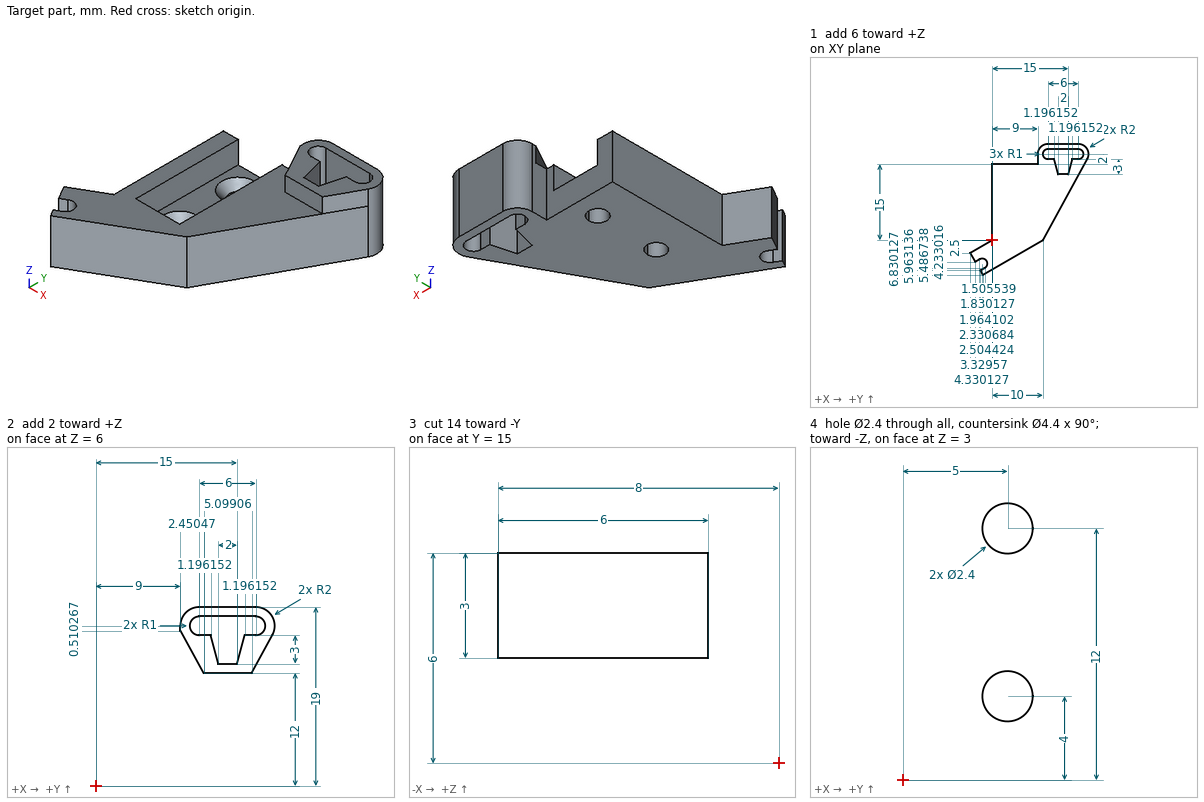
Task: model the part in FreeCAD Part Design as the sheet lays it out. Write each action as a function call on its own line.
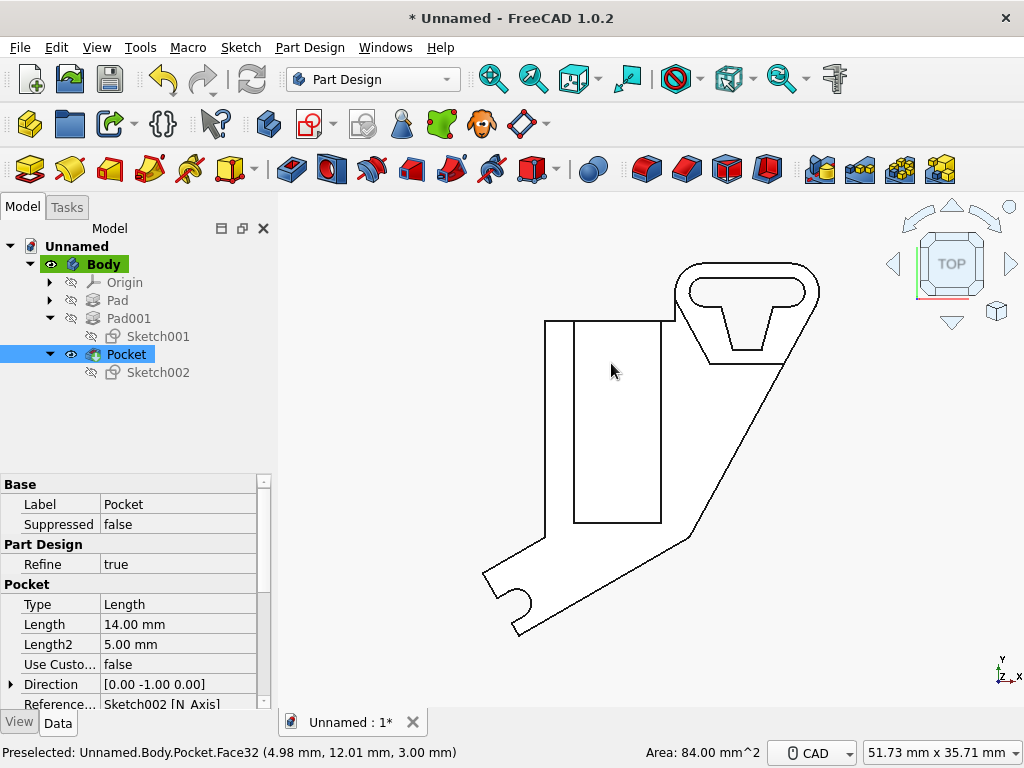
click(310, 124)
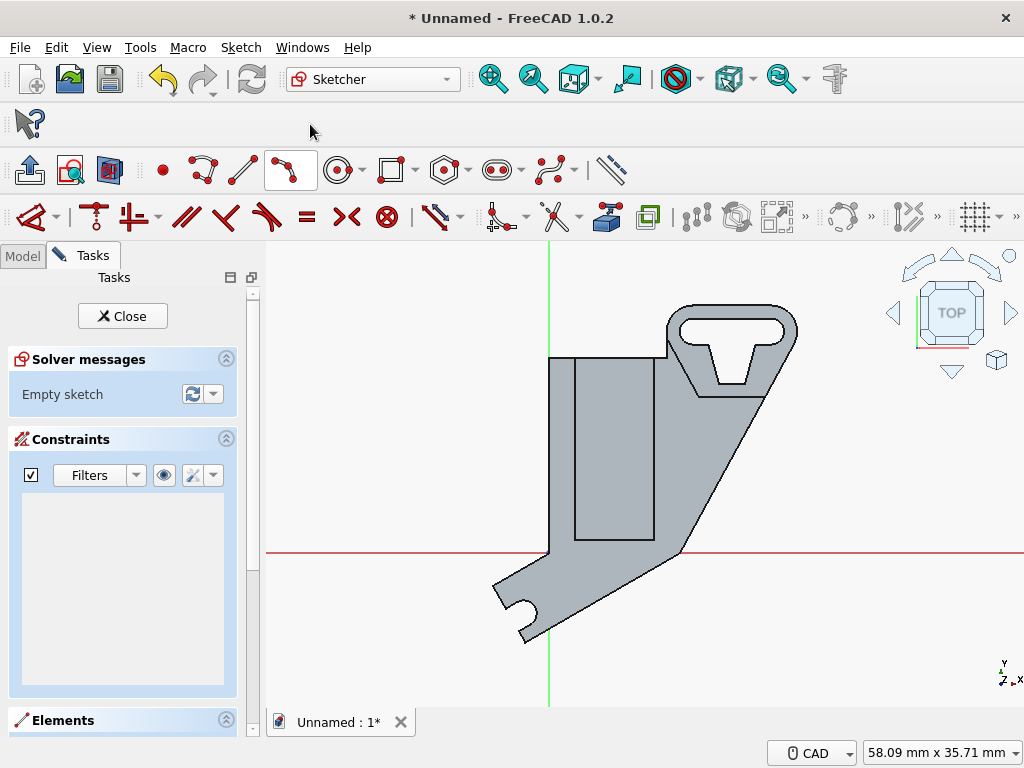
click(110, 170)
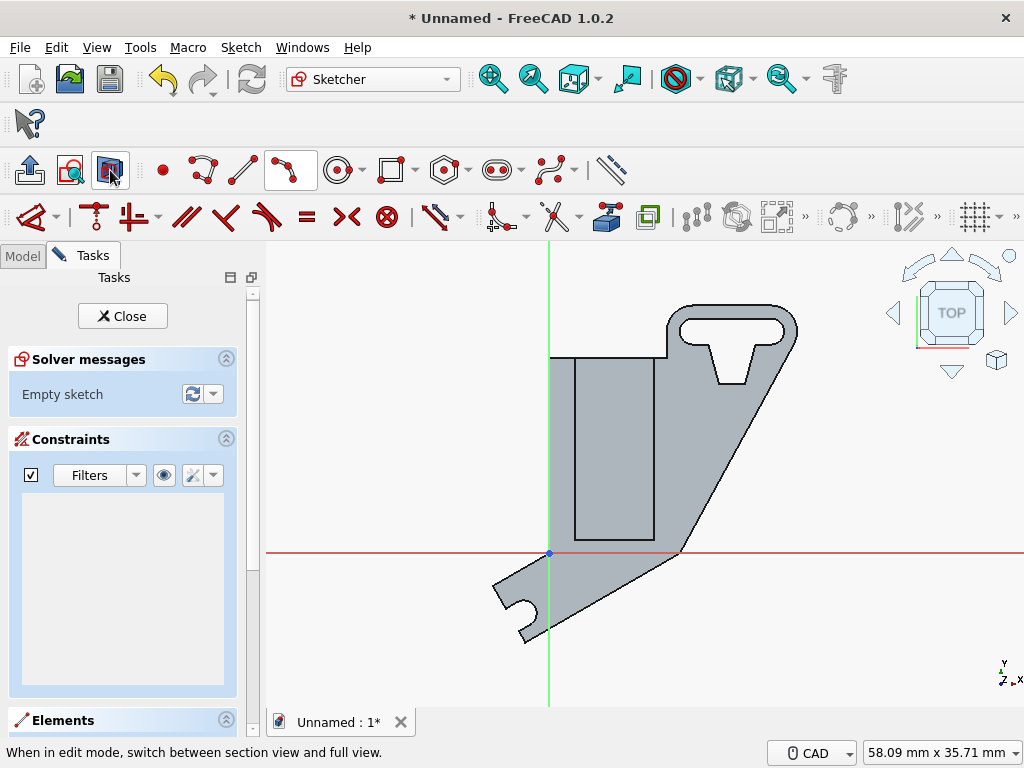
scroll(606, 459, up, 3)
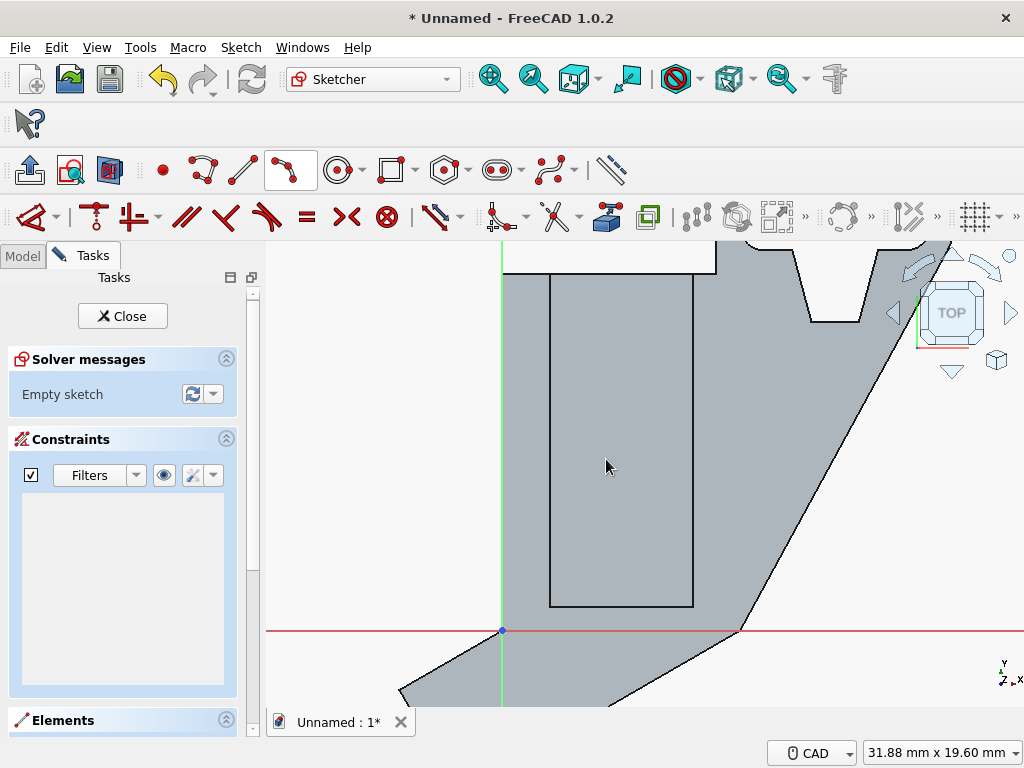
click(338, 170)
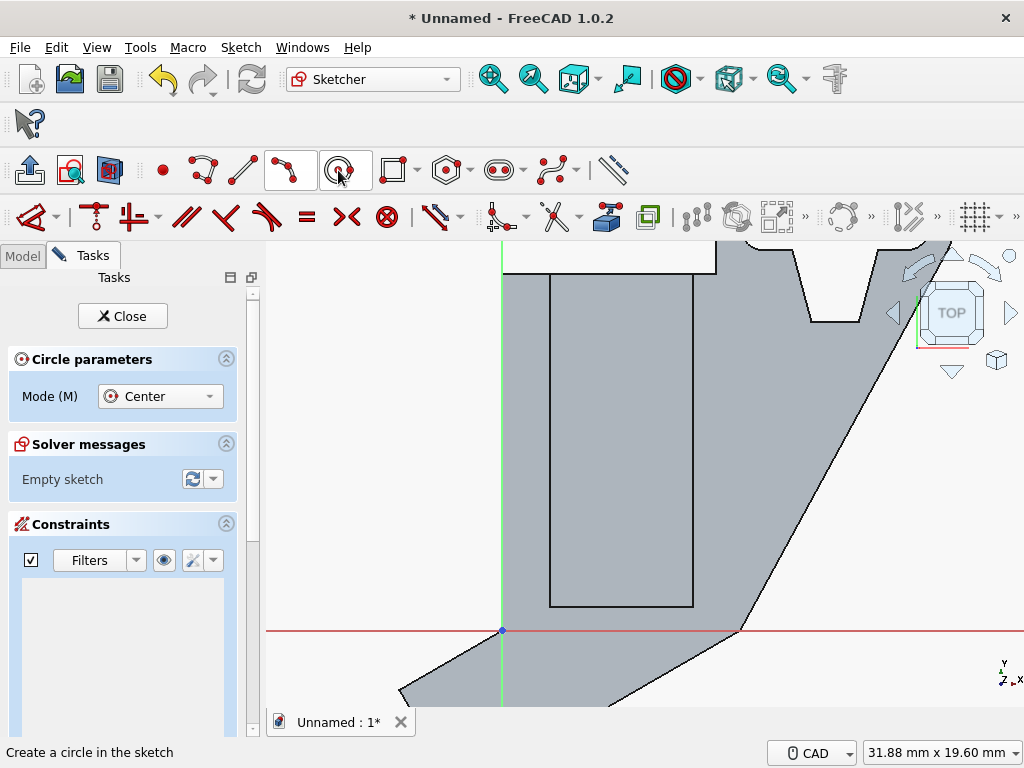
click(621, 345)
click(641, 325)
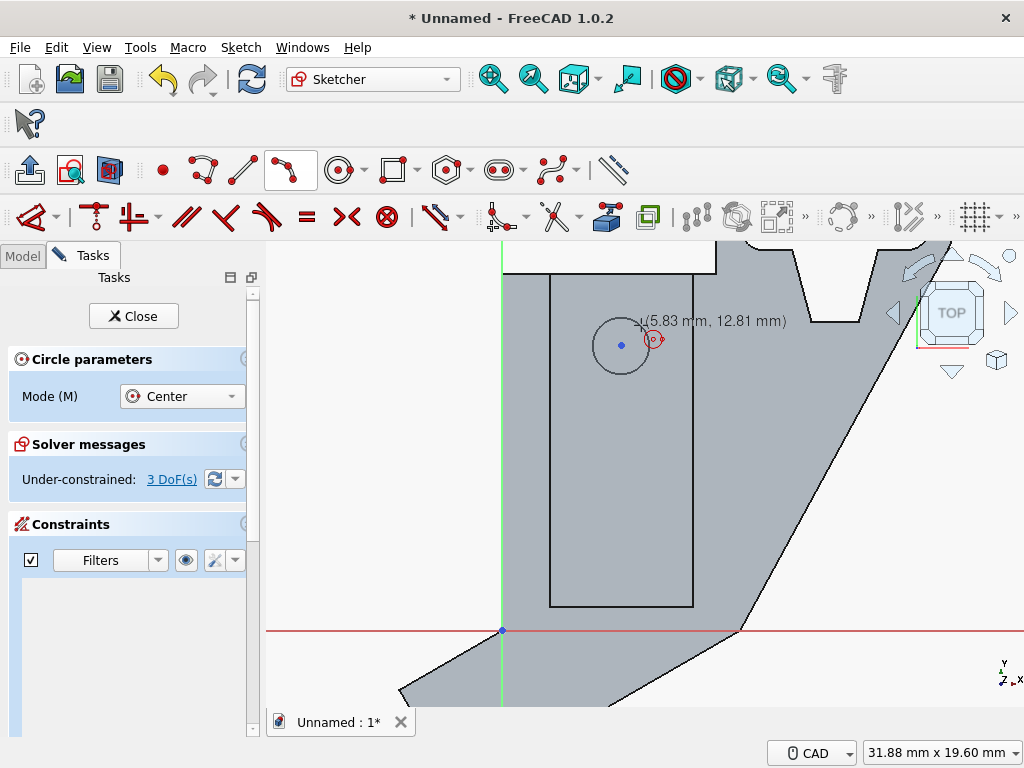
click(621, 536)
click(641, 515)
key(Escape)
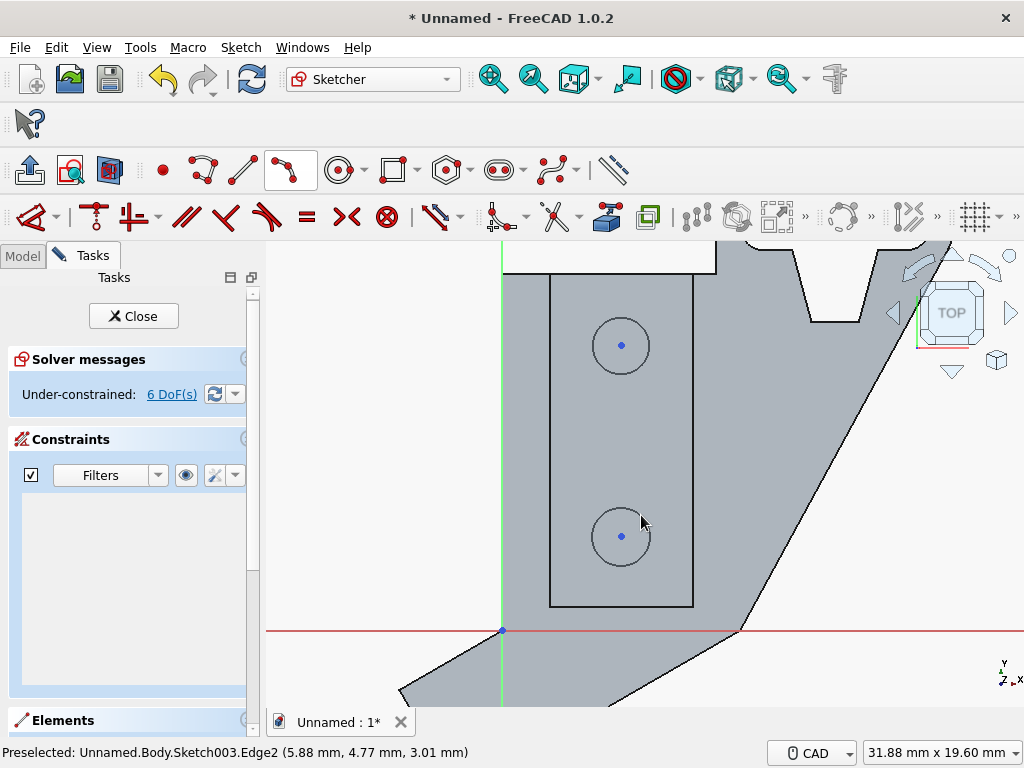
click(641, 326)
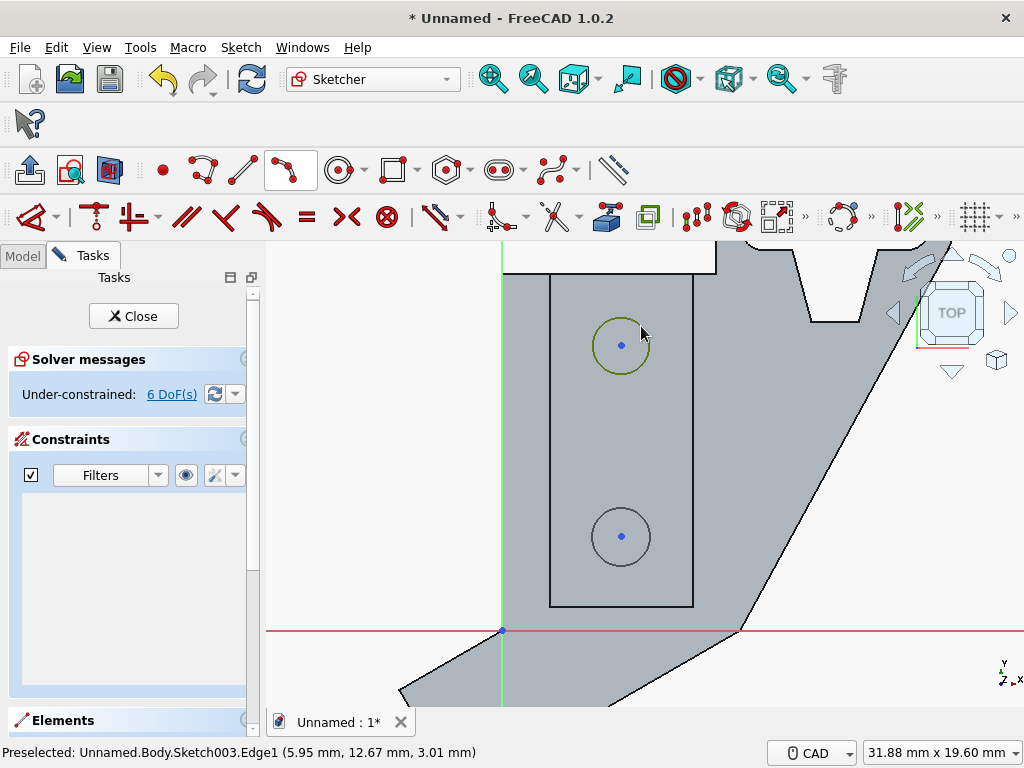
click(641, 516)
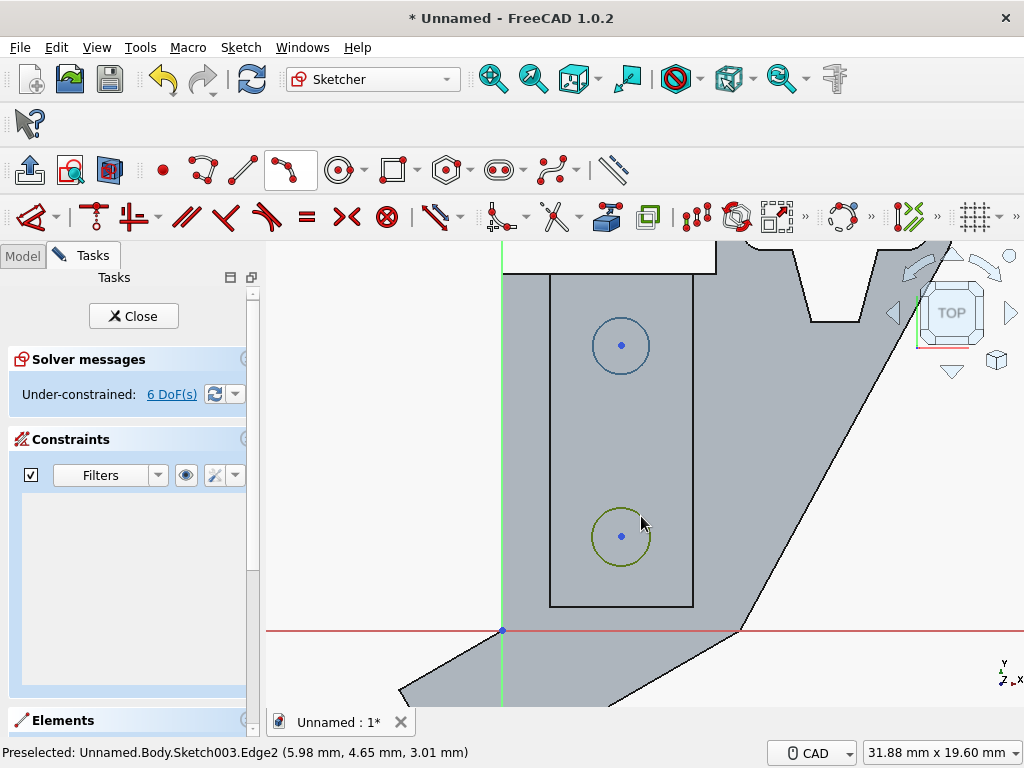
key(e)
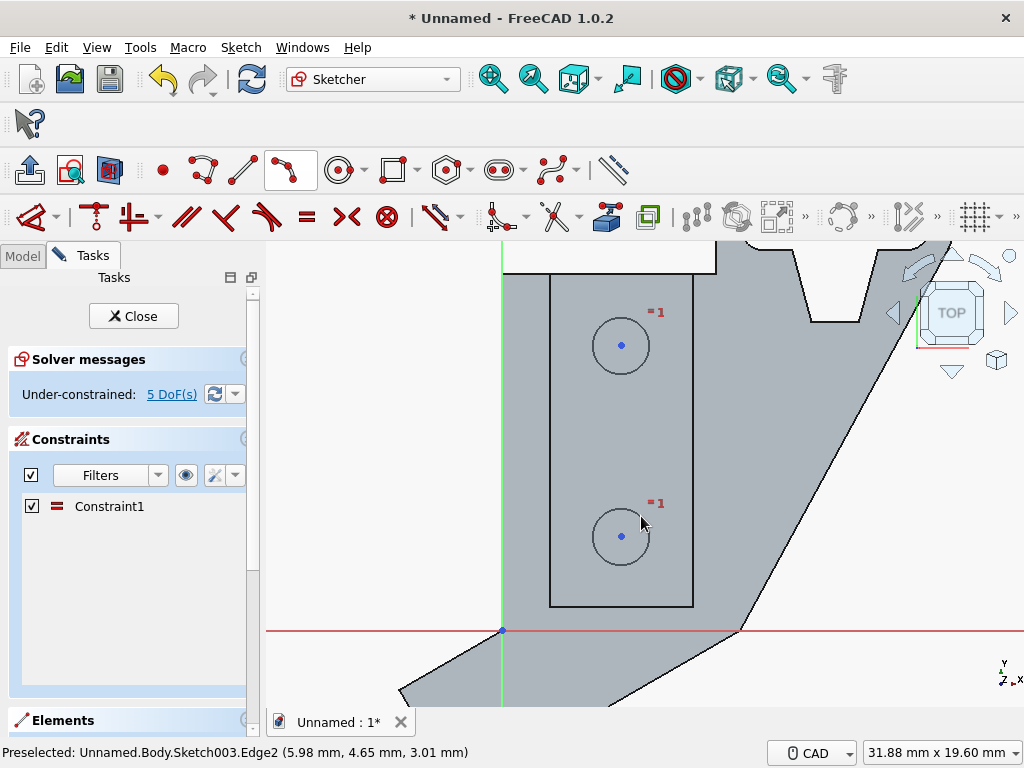
click(621, 346)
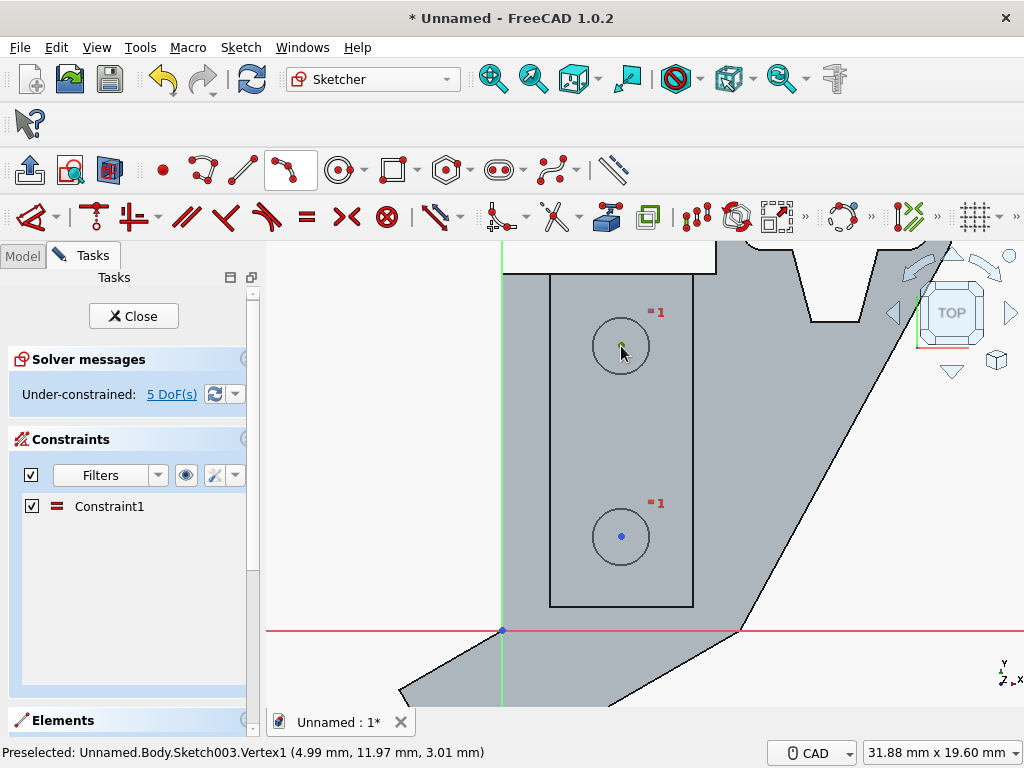
click(621, 537)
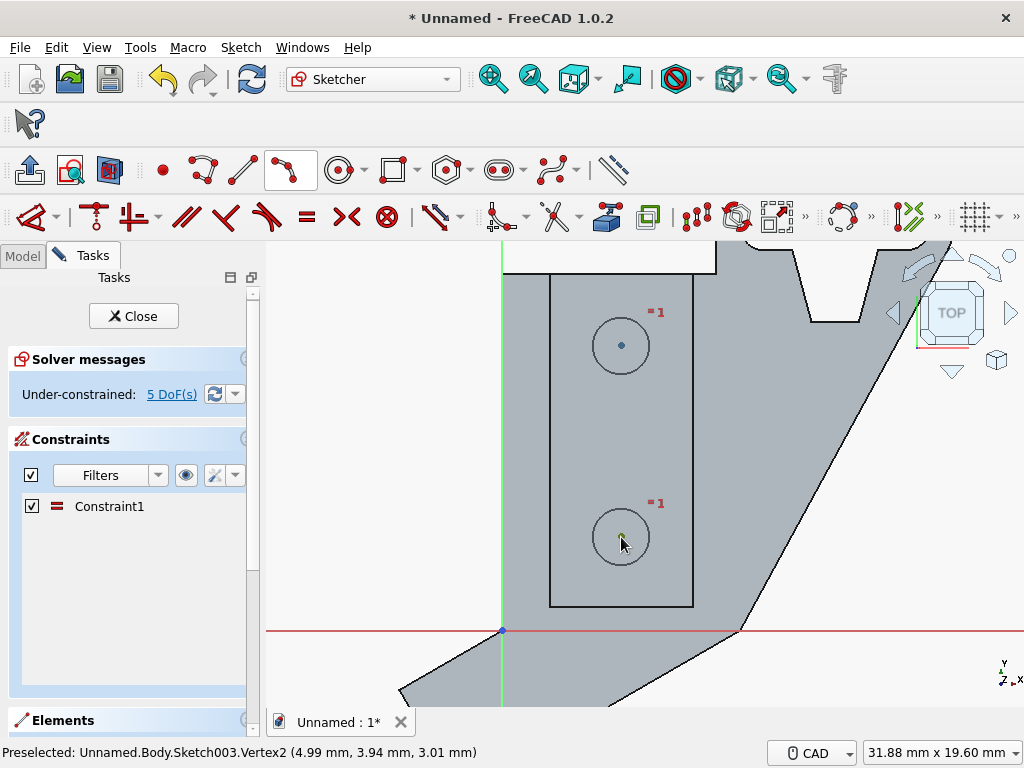
key(v)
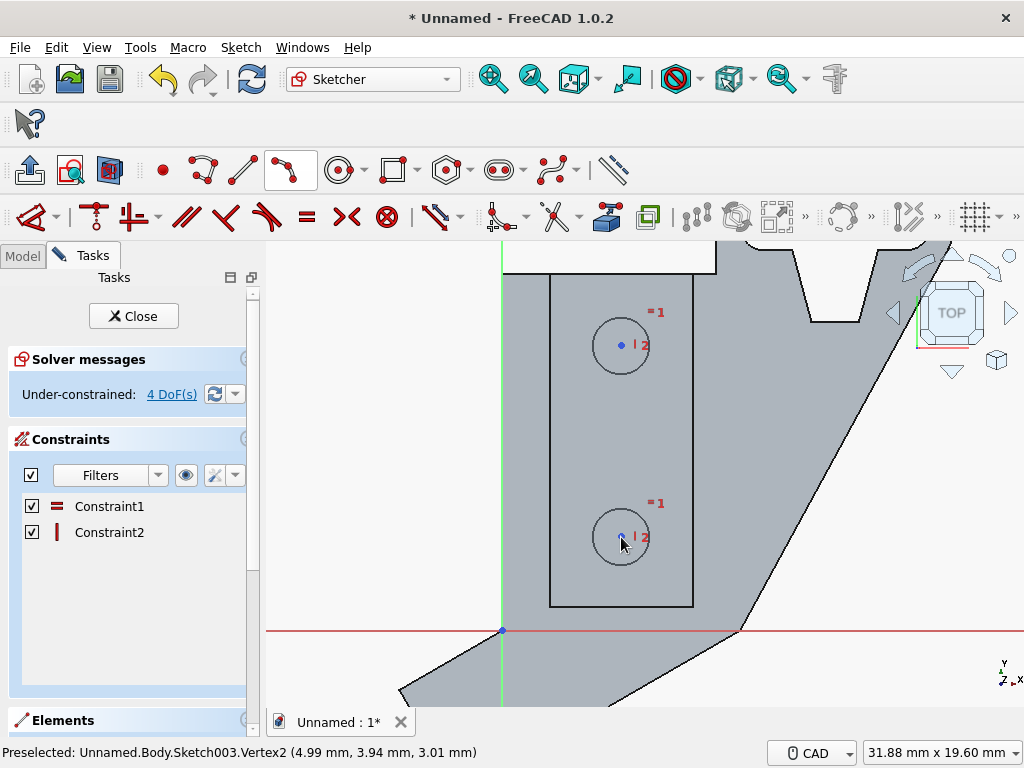
key(d)